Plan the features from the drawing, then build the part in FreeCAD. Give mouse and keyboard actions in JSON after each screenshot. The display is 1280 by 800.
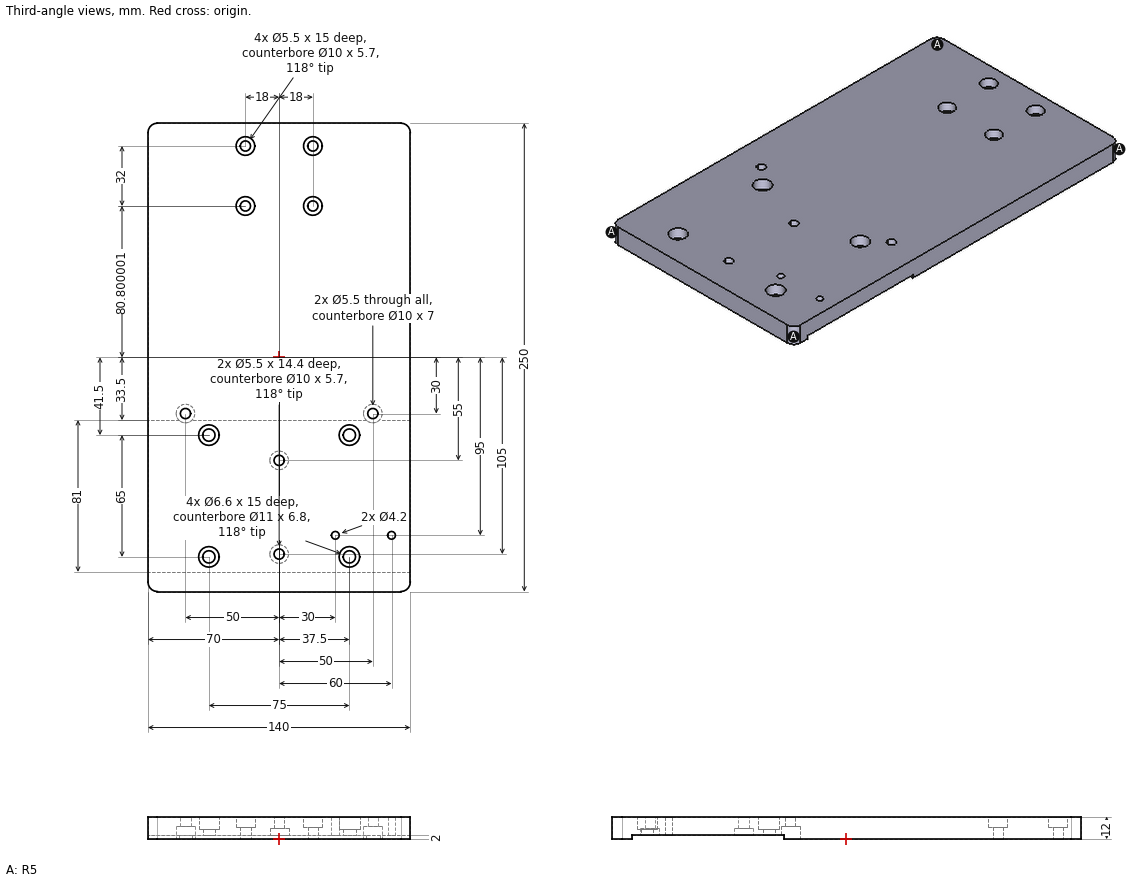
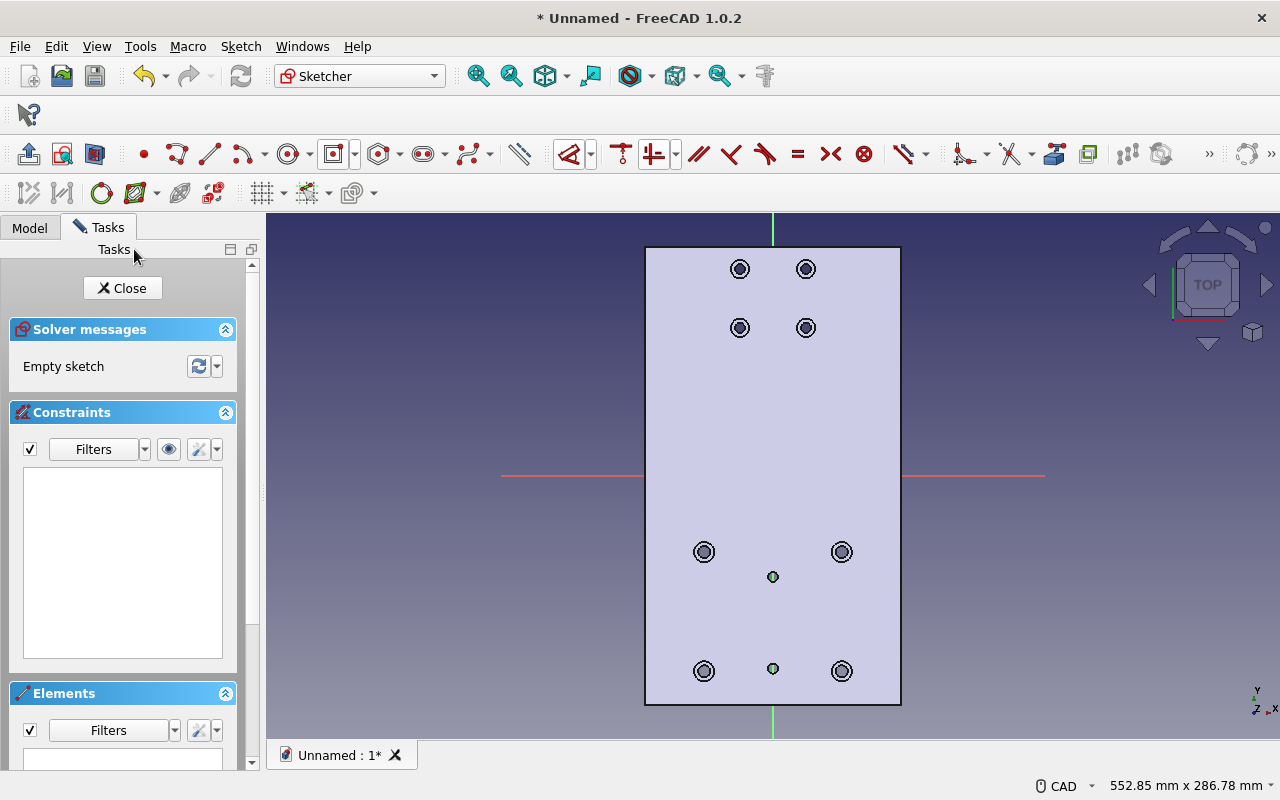
{"action": "left_click", "coordinate": [95, 154]}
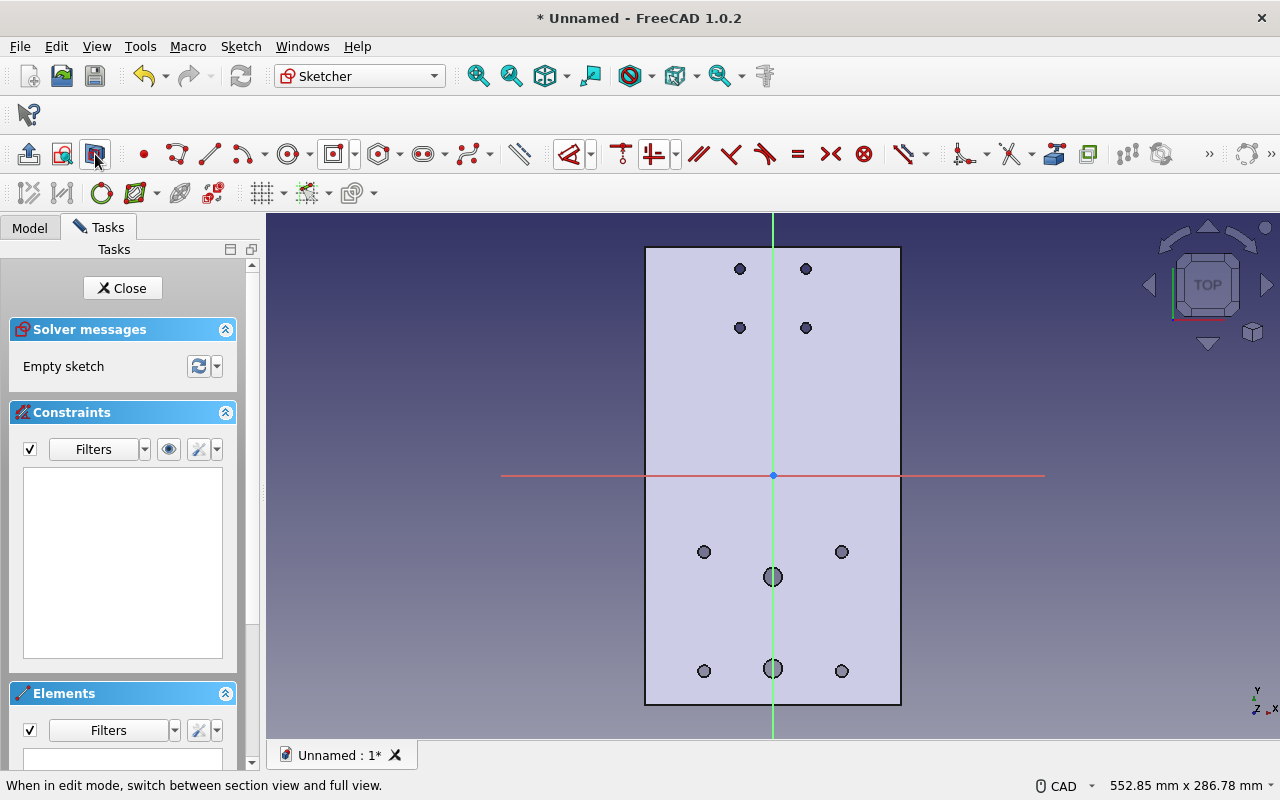
{"action": "scroll", "coordinate": [912, 711], "scroll_direction": "up", "scroll_amount": 2}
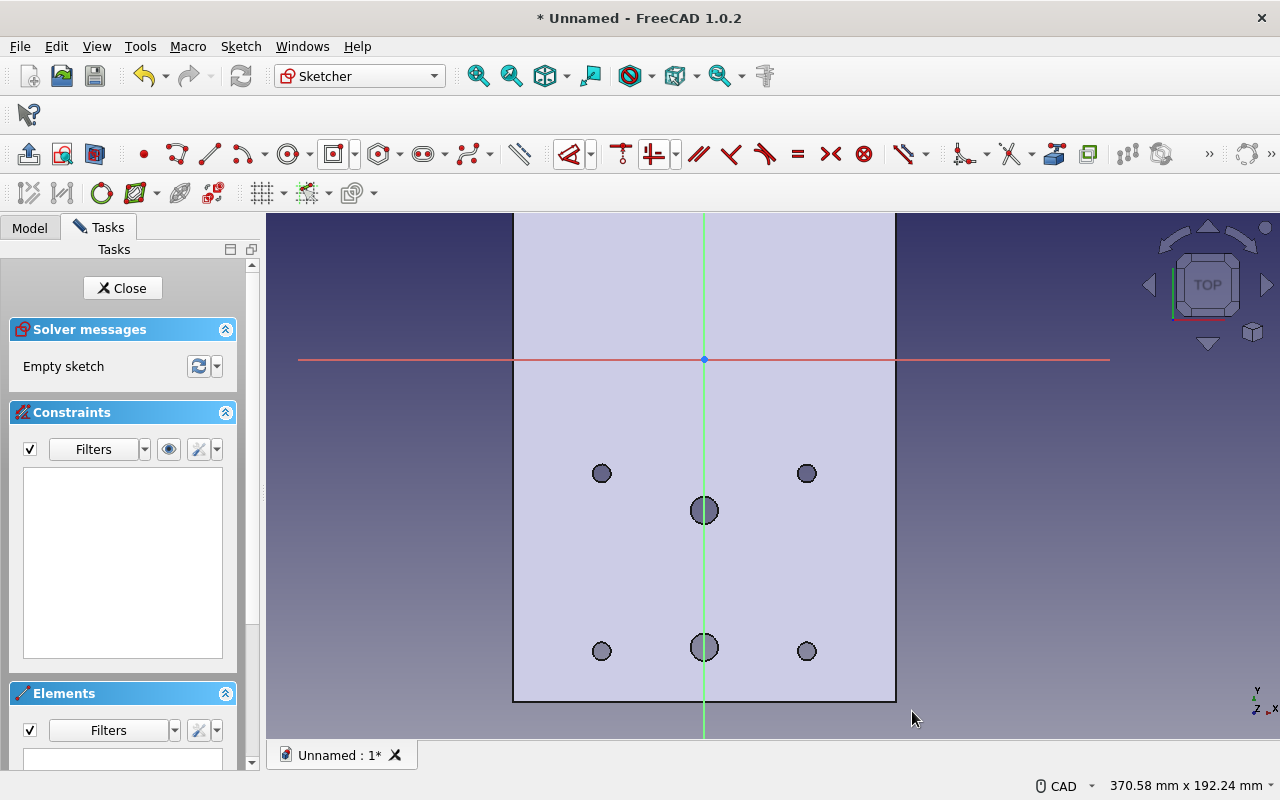
{"action": "key", "text": "g r"}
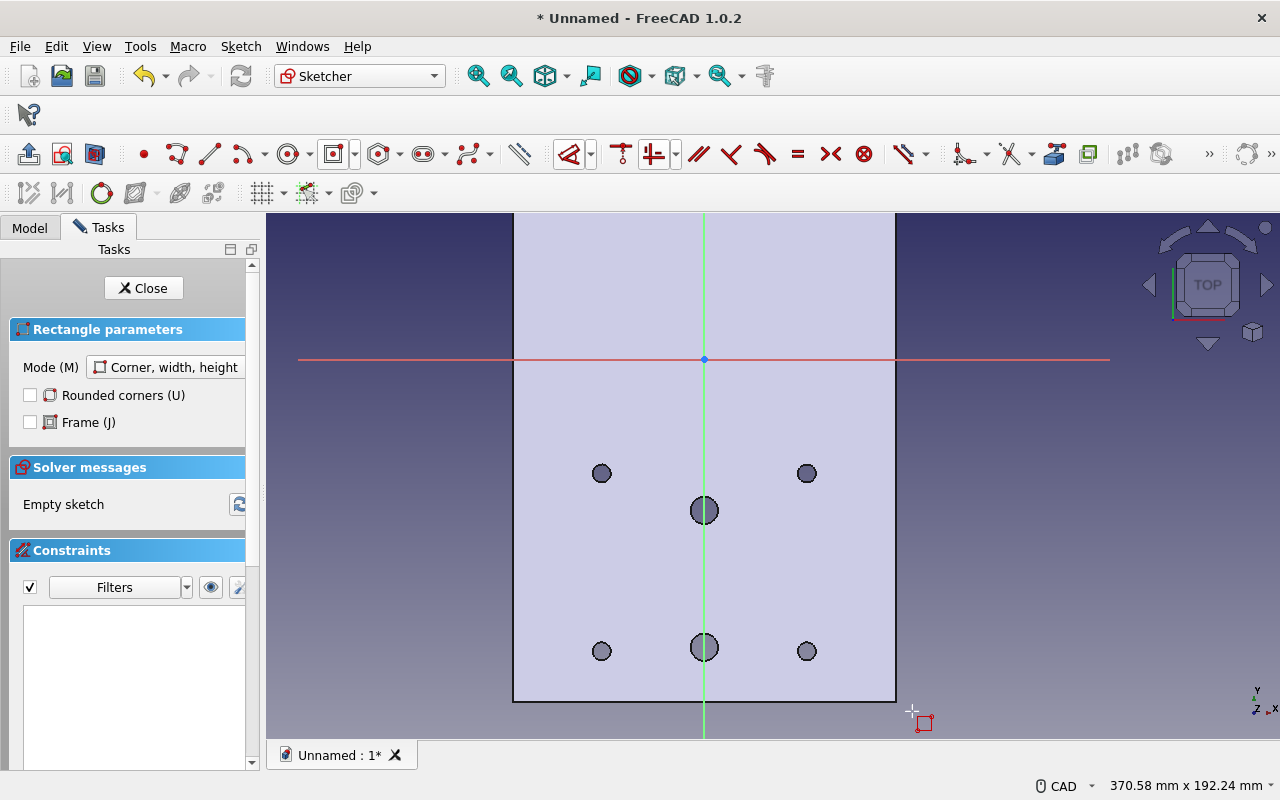
{"action": "left_click", "coordinate": [513, 452]}
{"action": "left_click", "coordinate": [896, 673]}
{"action": "key", "text": "Escape"}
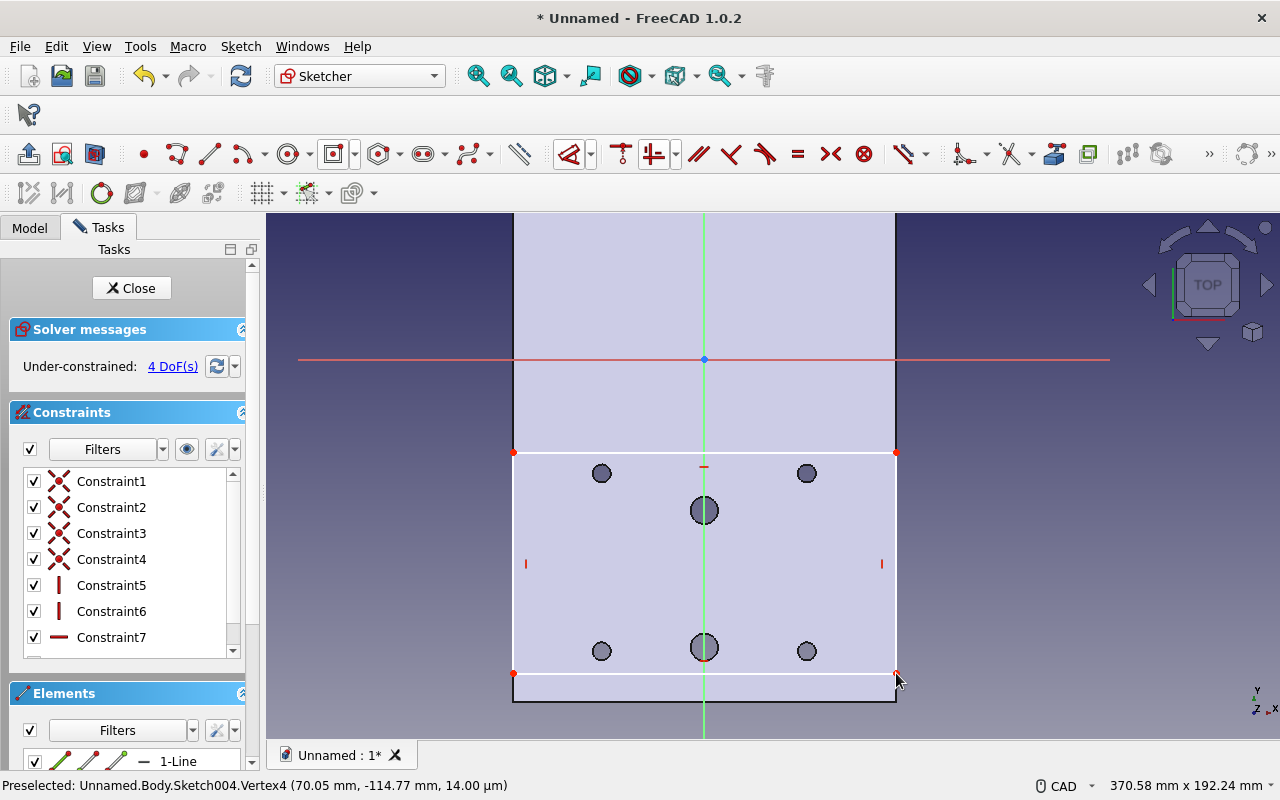
{"action": "left_click", "coordinate": [513, 519]}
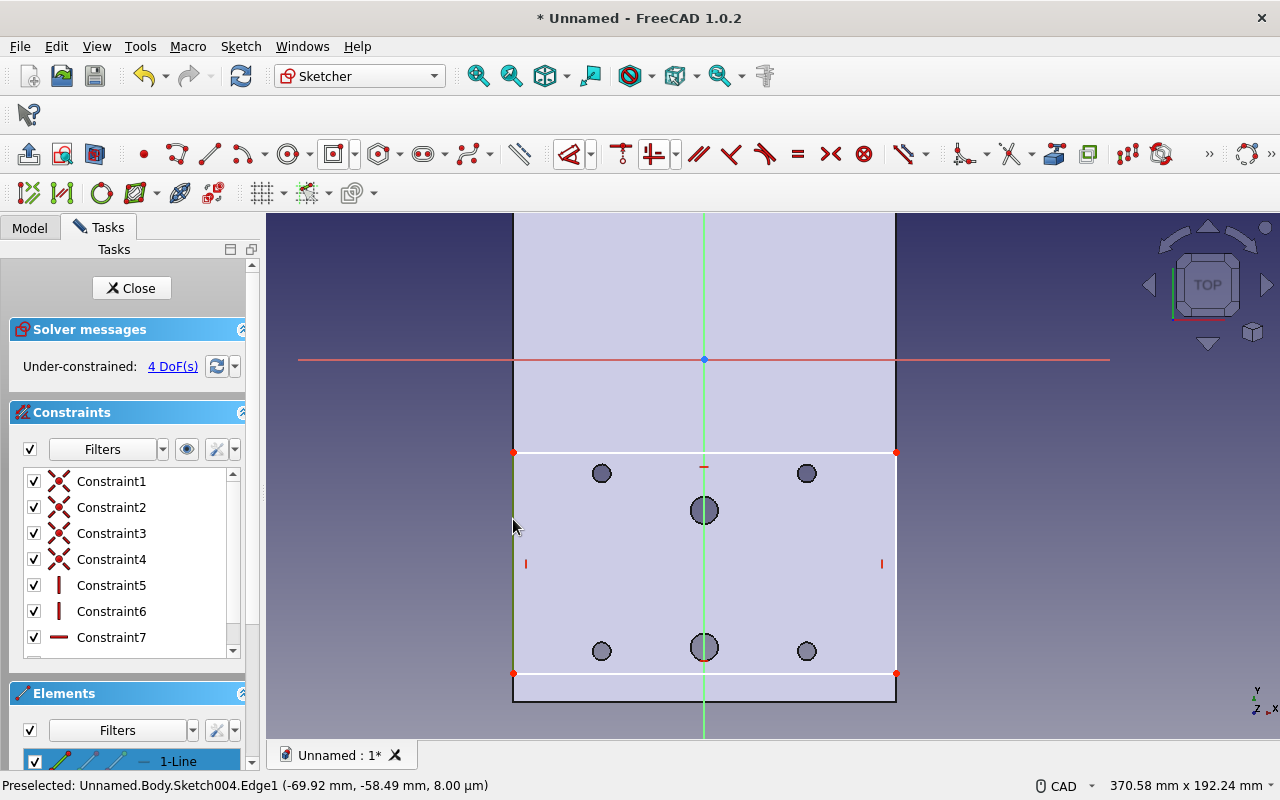
{"action": "key", "text": "i"}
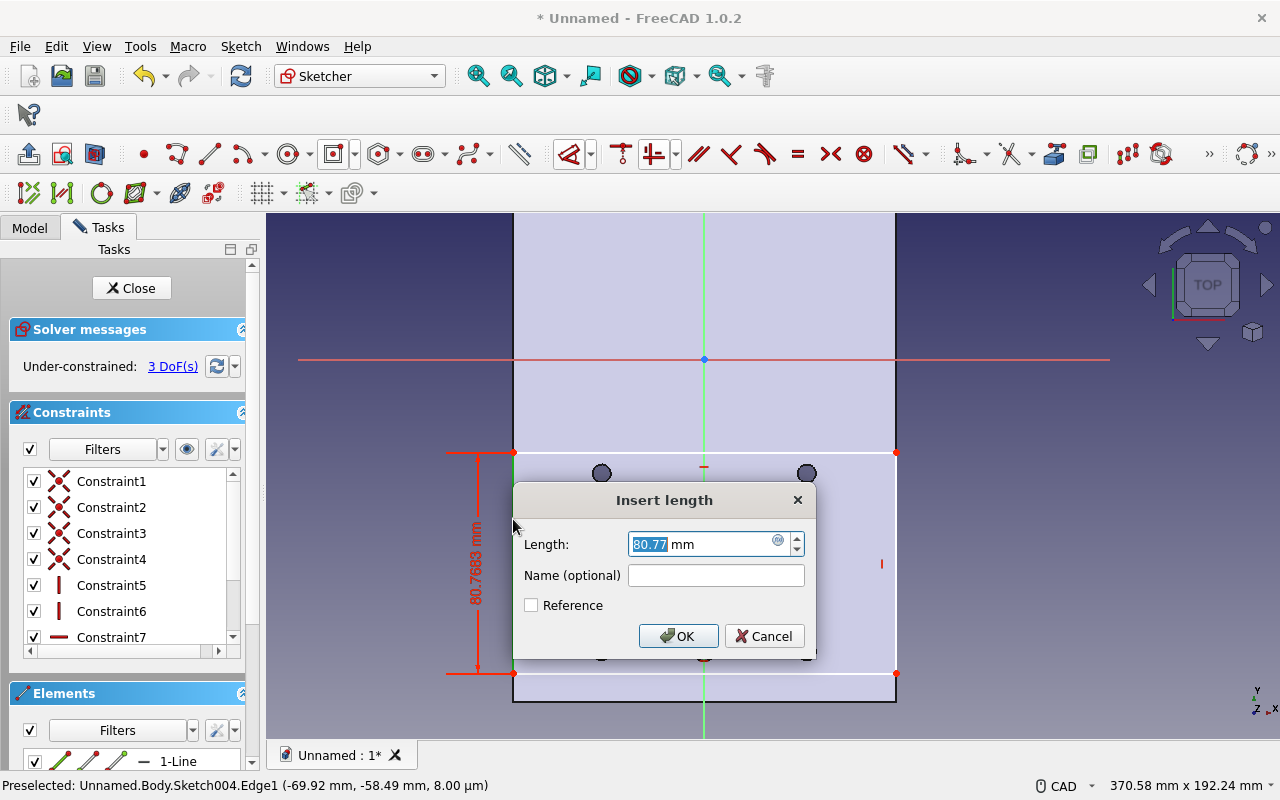
{"action": "type", "text": "81"}
{"action": "key", "text": "Return"}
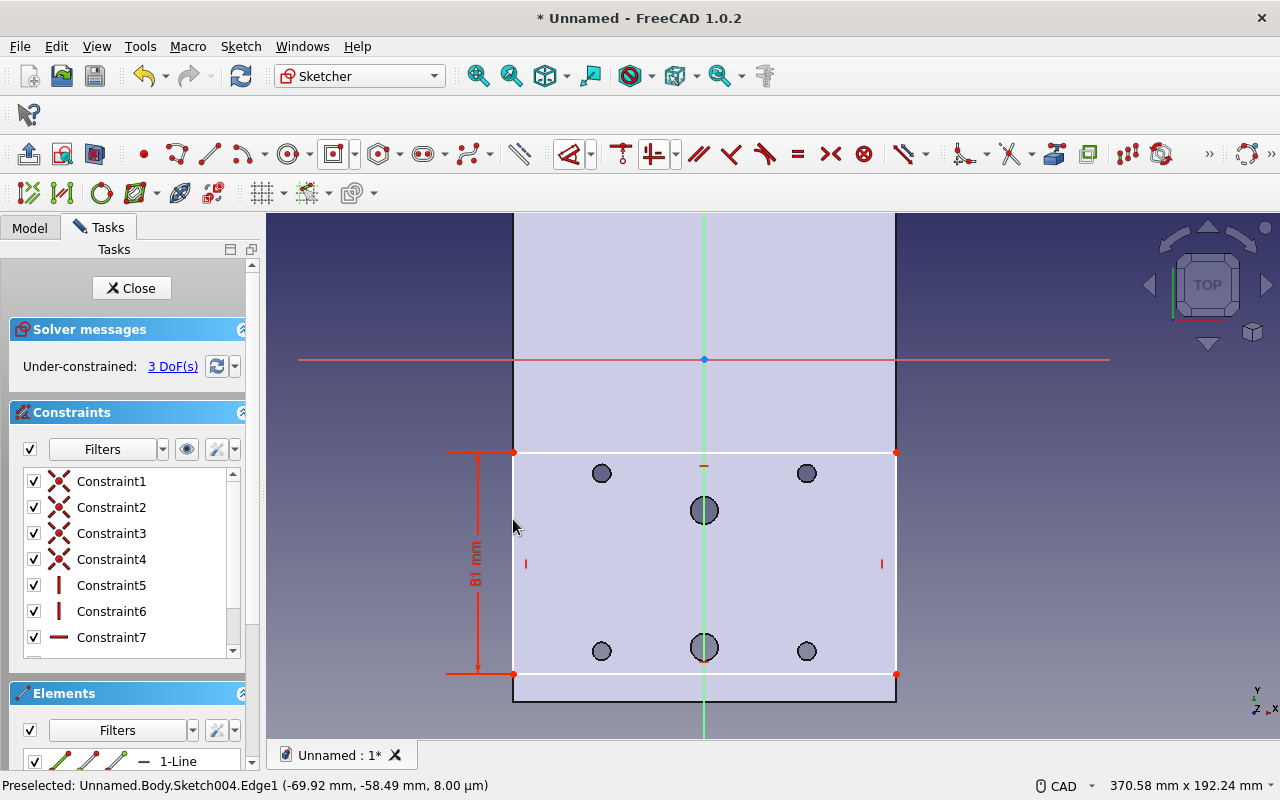
{"action": "left_click", "coordinate": [628, 674]}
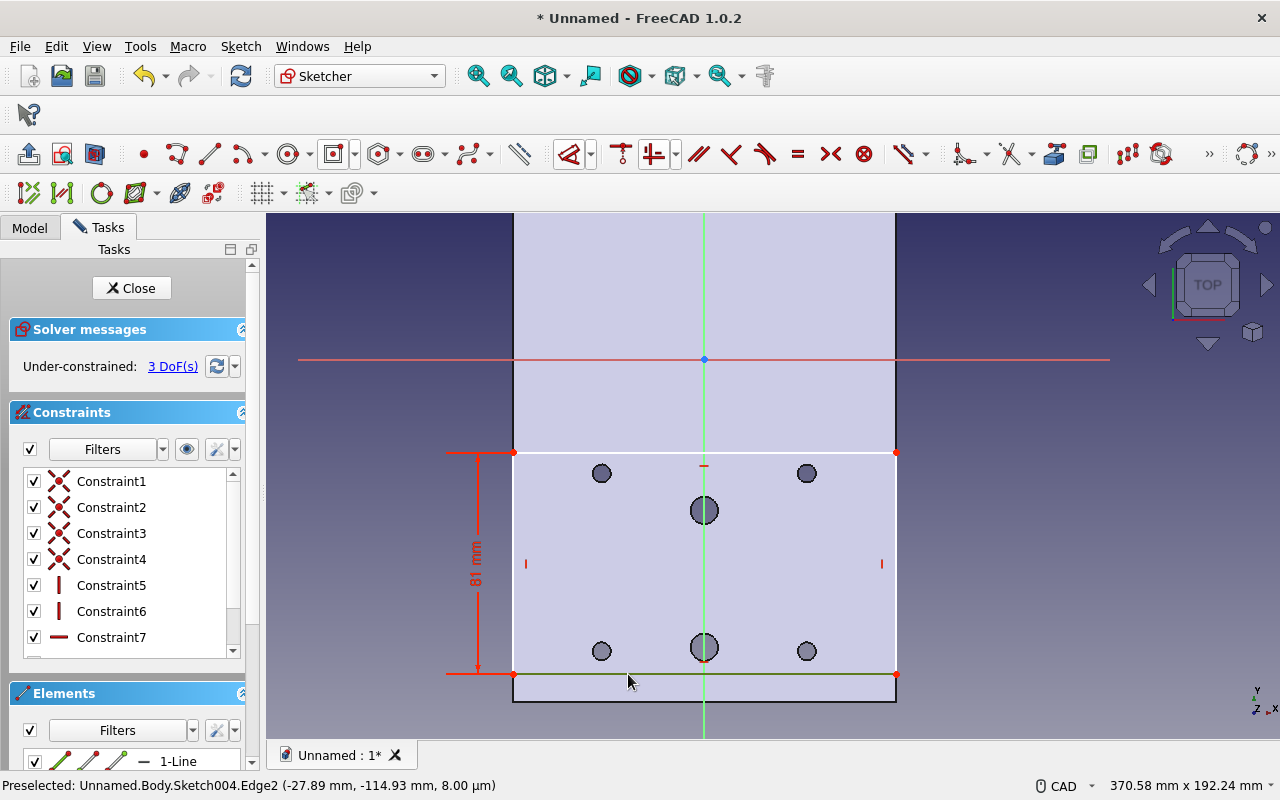
{"action": "key", "text": "l"}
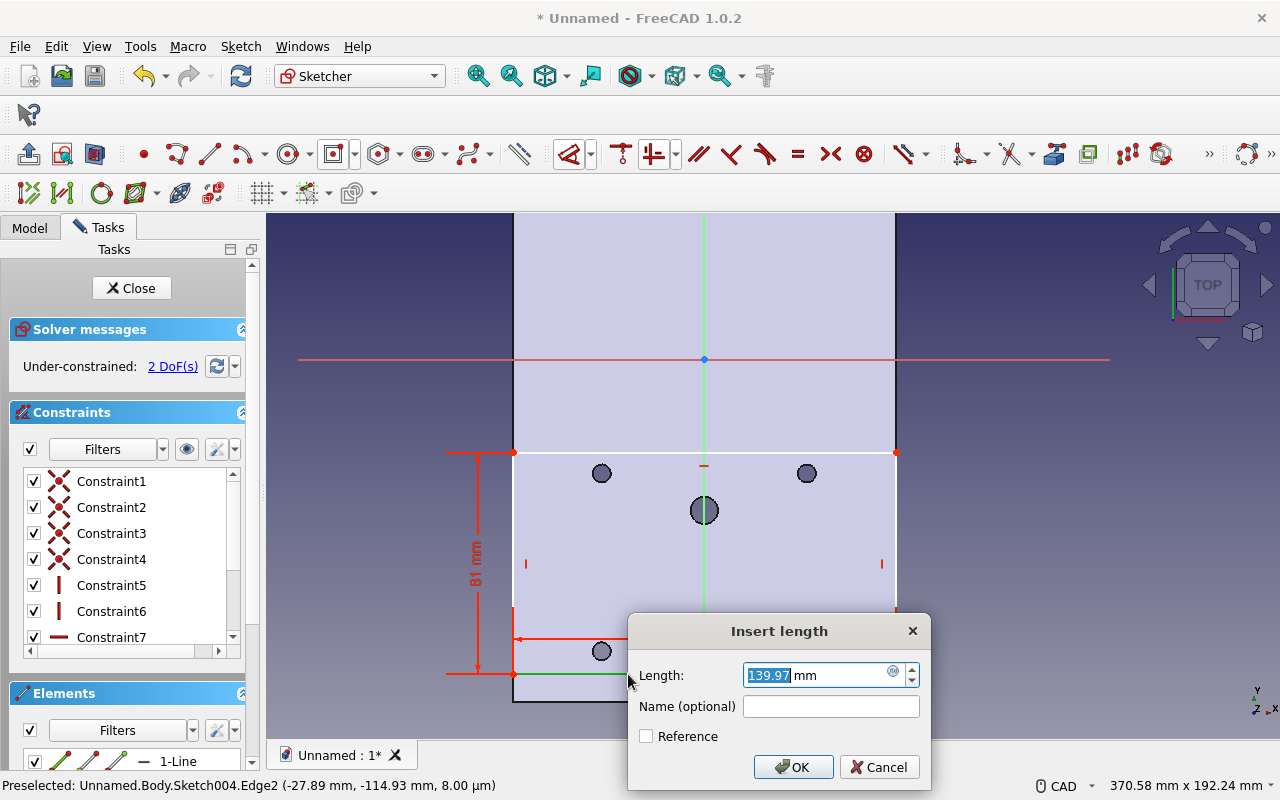
{"action": "type", "text": "140"}
{"action": "key", "text": "Return"}